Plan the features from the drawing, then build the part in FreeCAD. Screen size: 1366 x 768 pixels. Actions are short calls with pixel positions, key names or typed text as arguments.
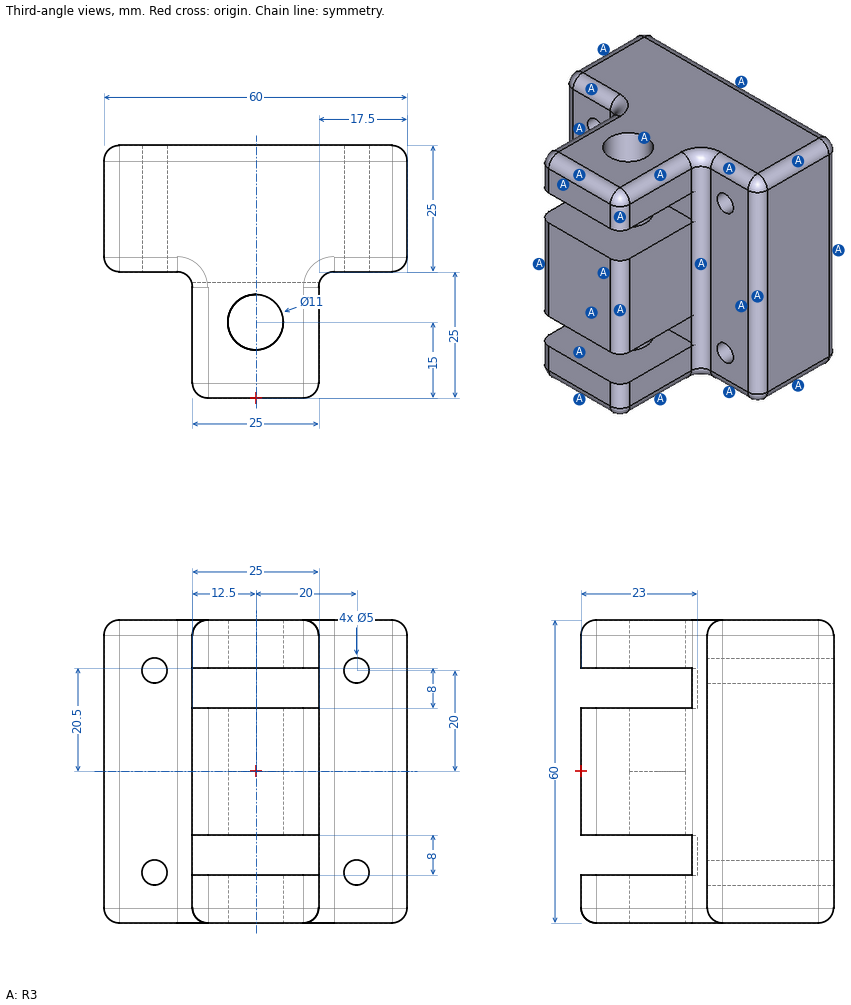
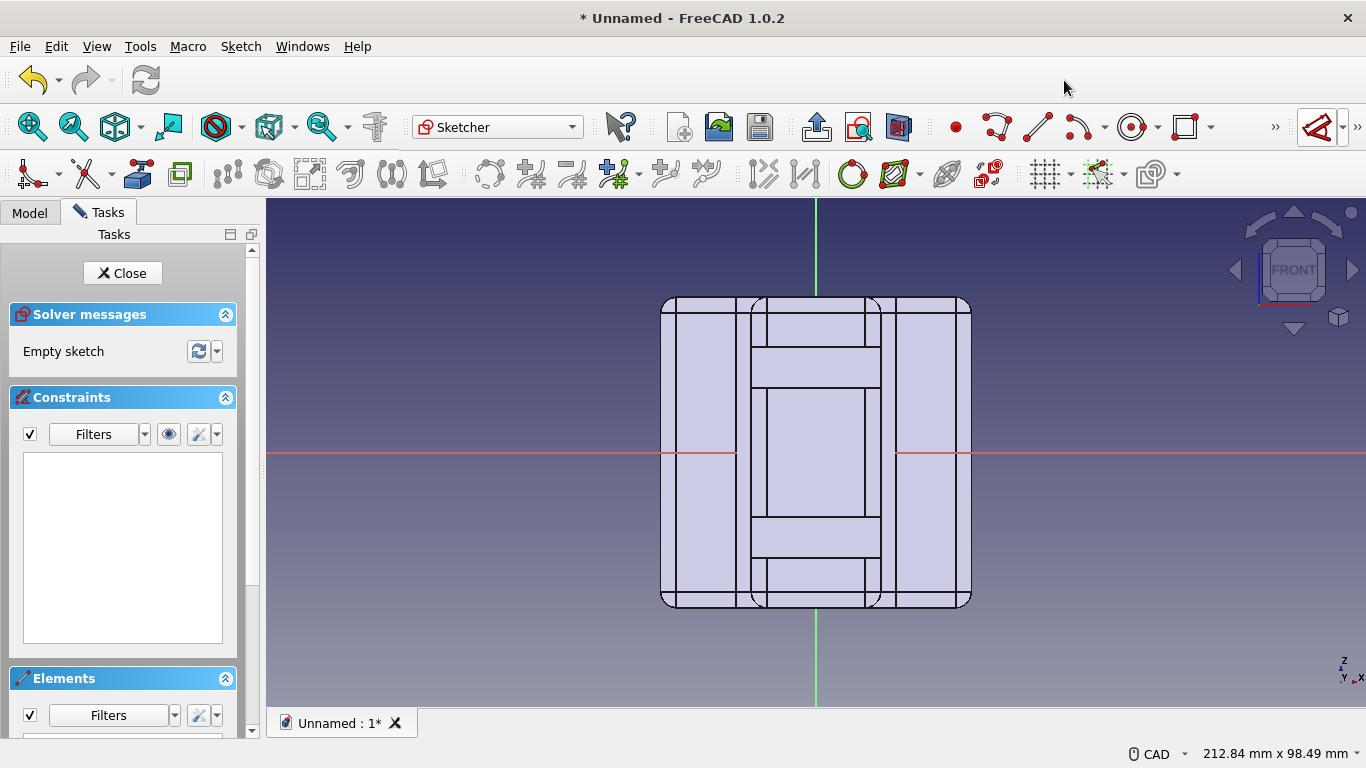
scroll(955, 453, up, 2)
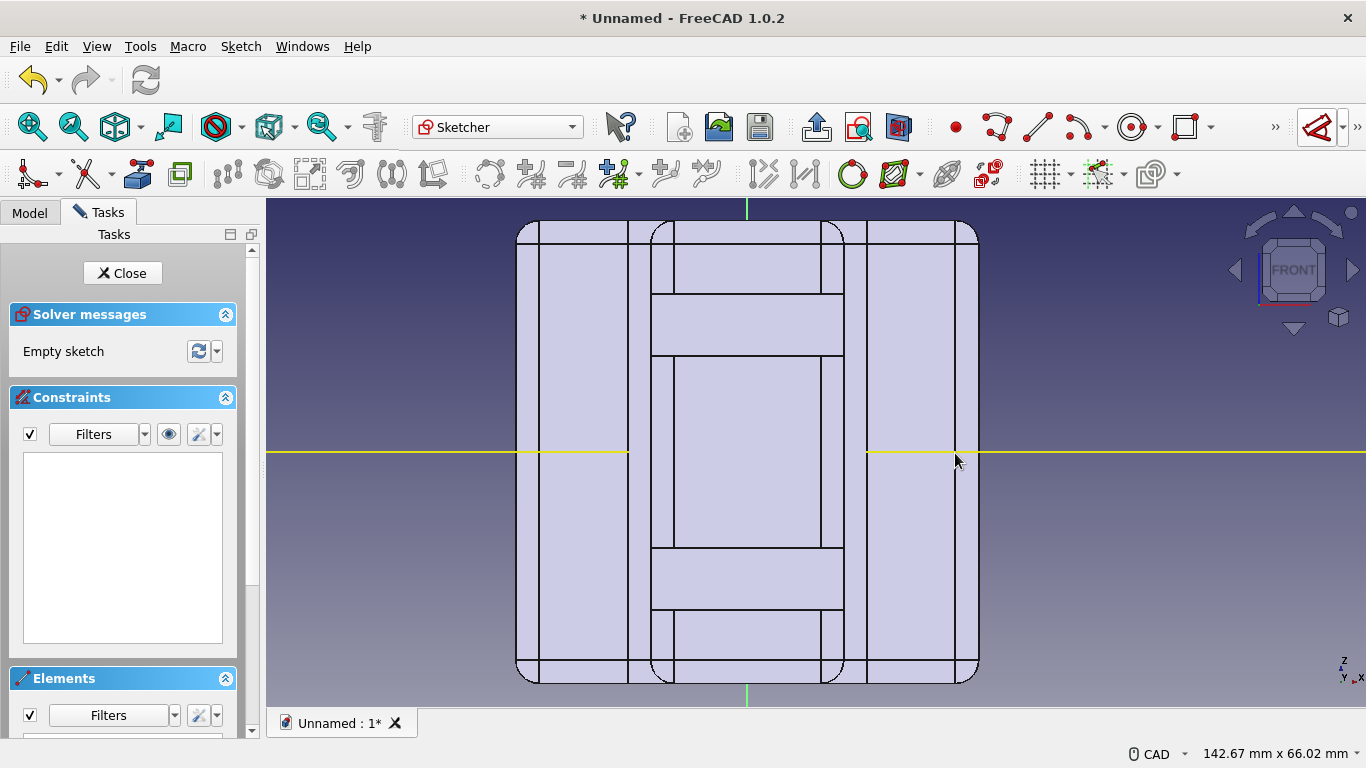
click(1132, 128)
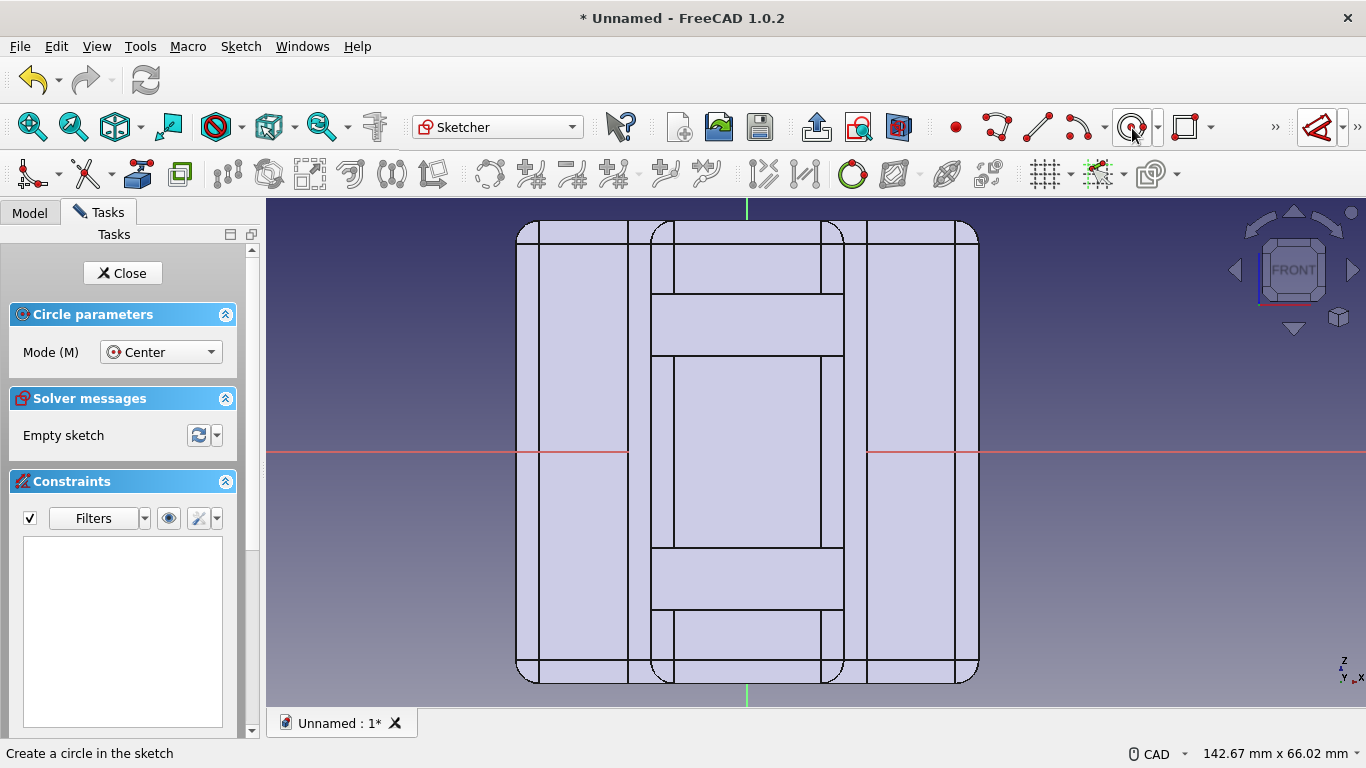
click(902, 298)
move(915, 284)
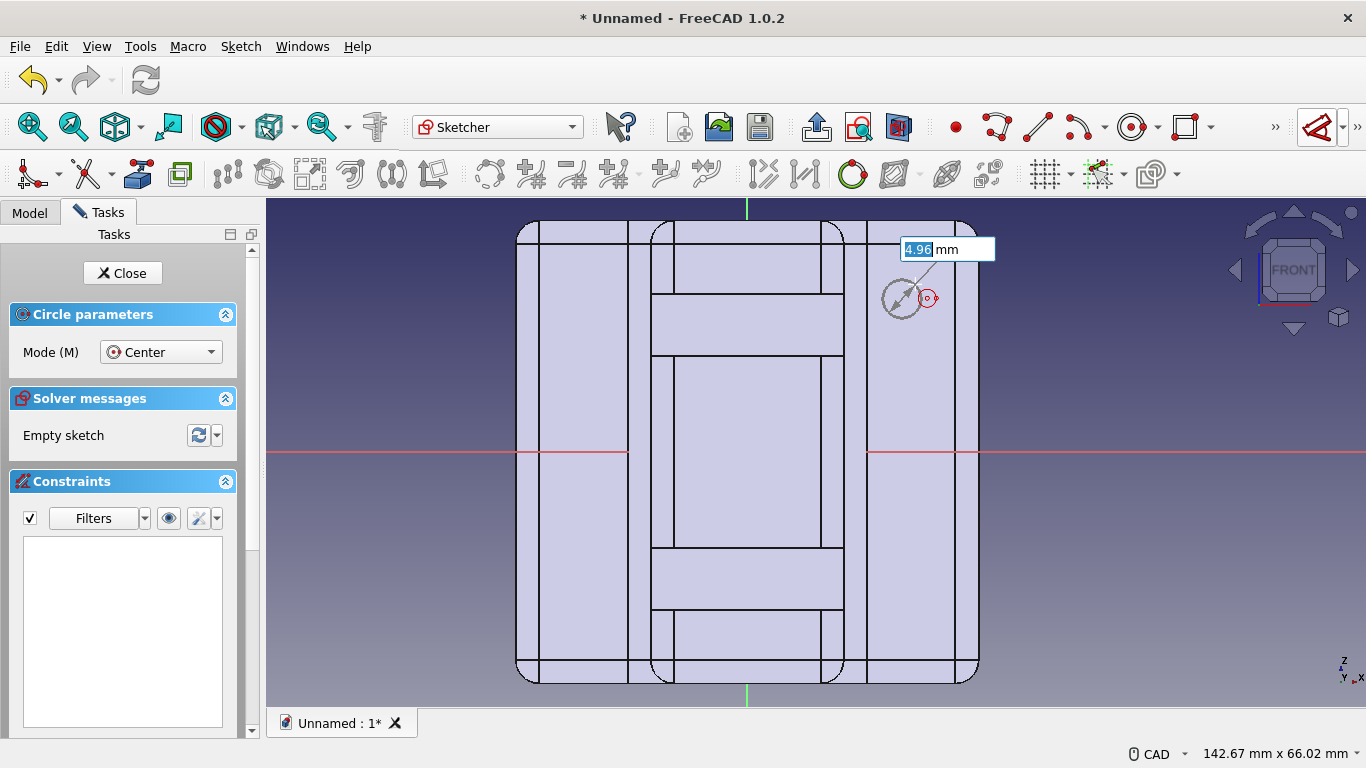
text(5)
key(Return)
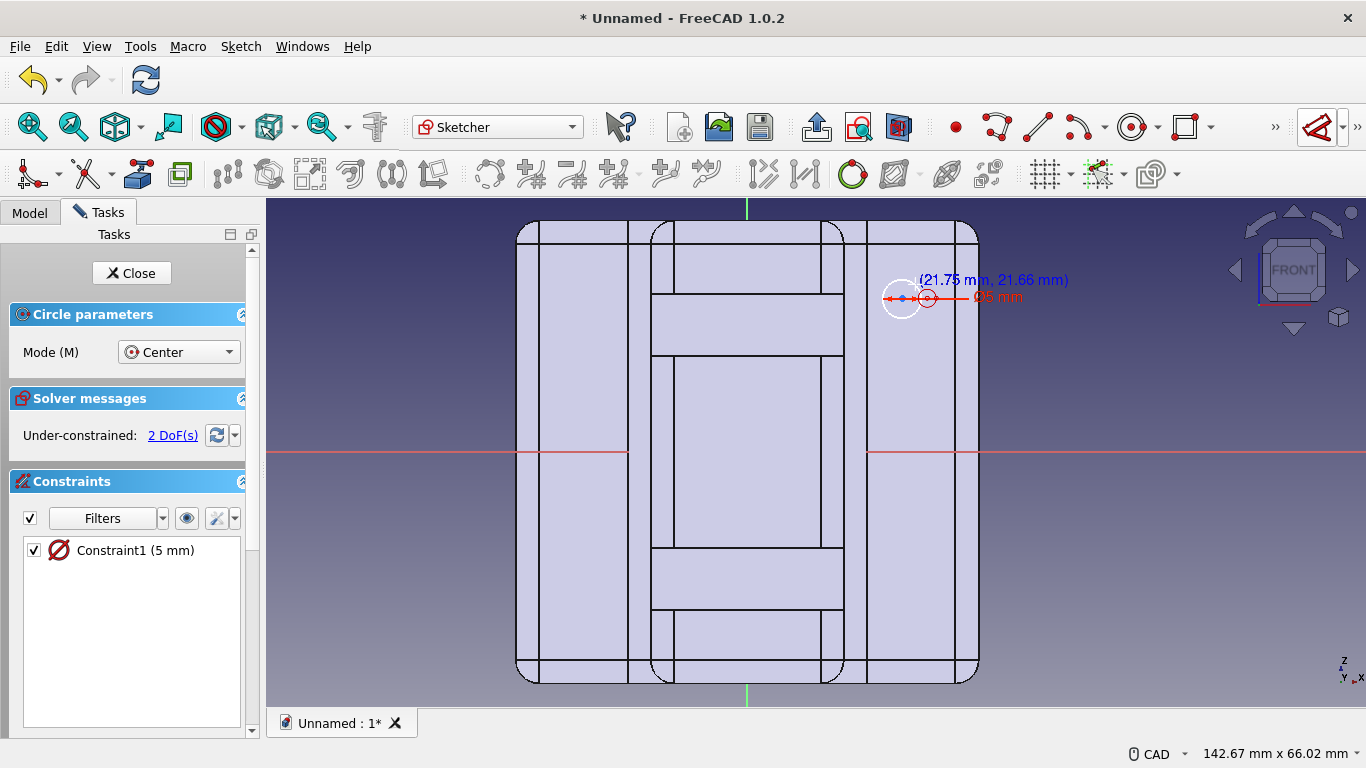
click(902, 606)
move(915, 593)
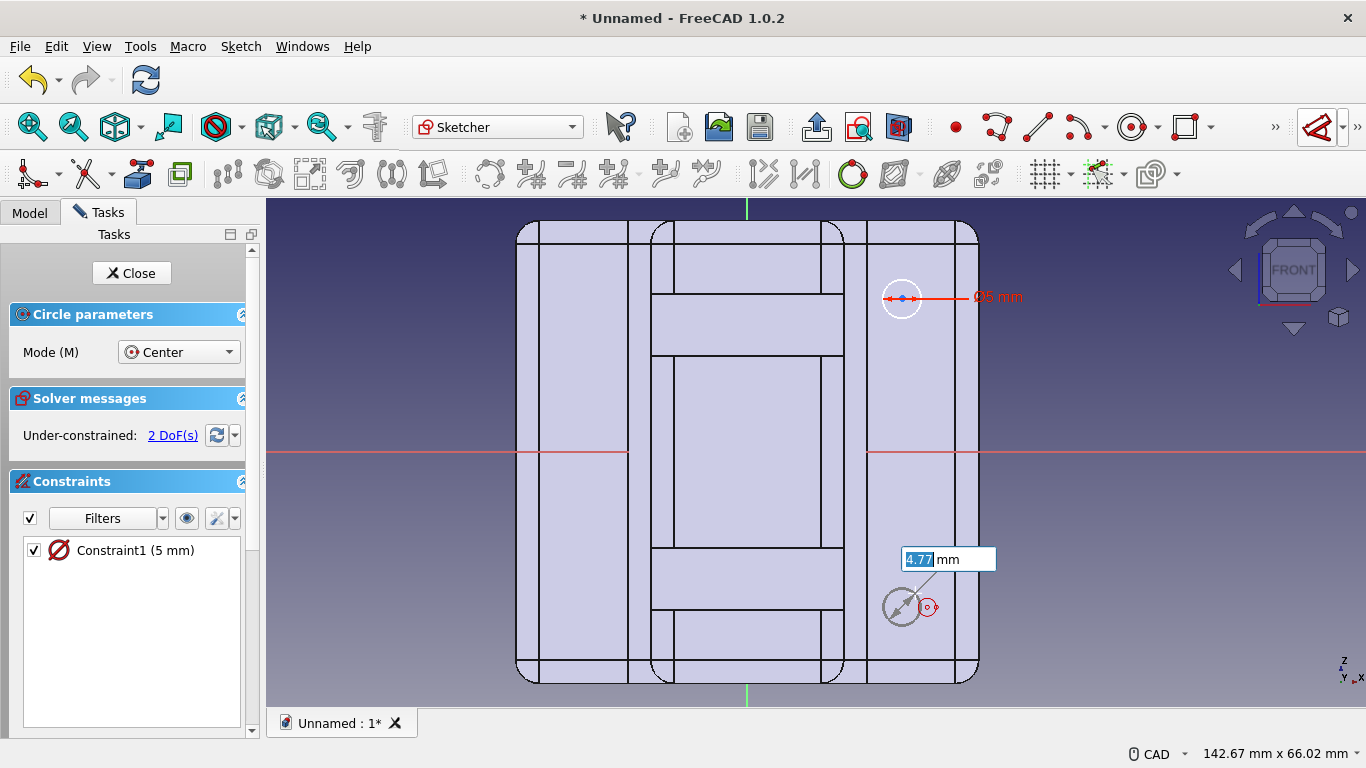
text(5)
key(Return)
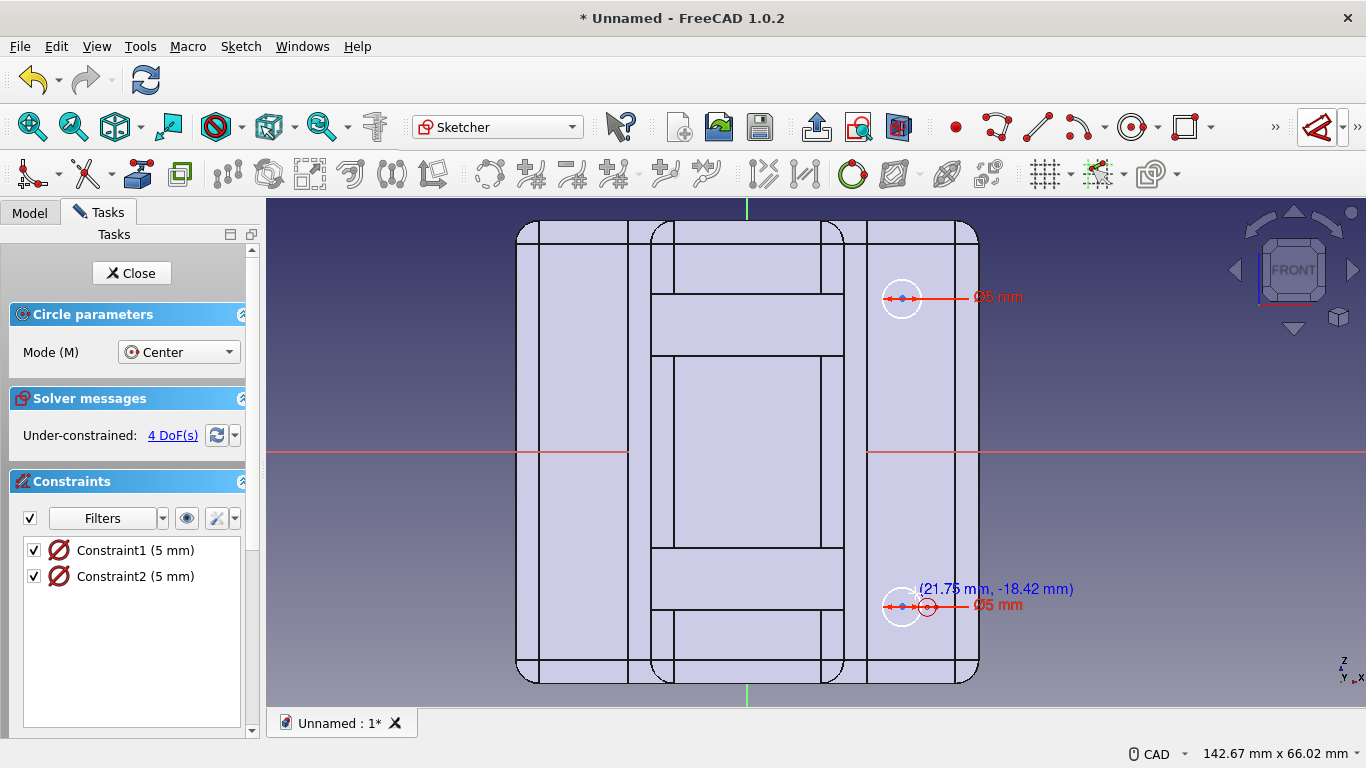
click(593, 606)
move(607, 593)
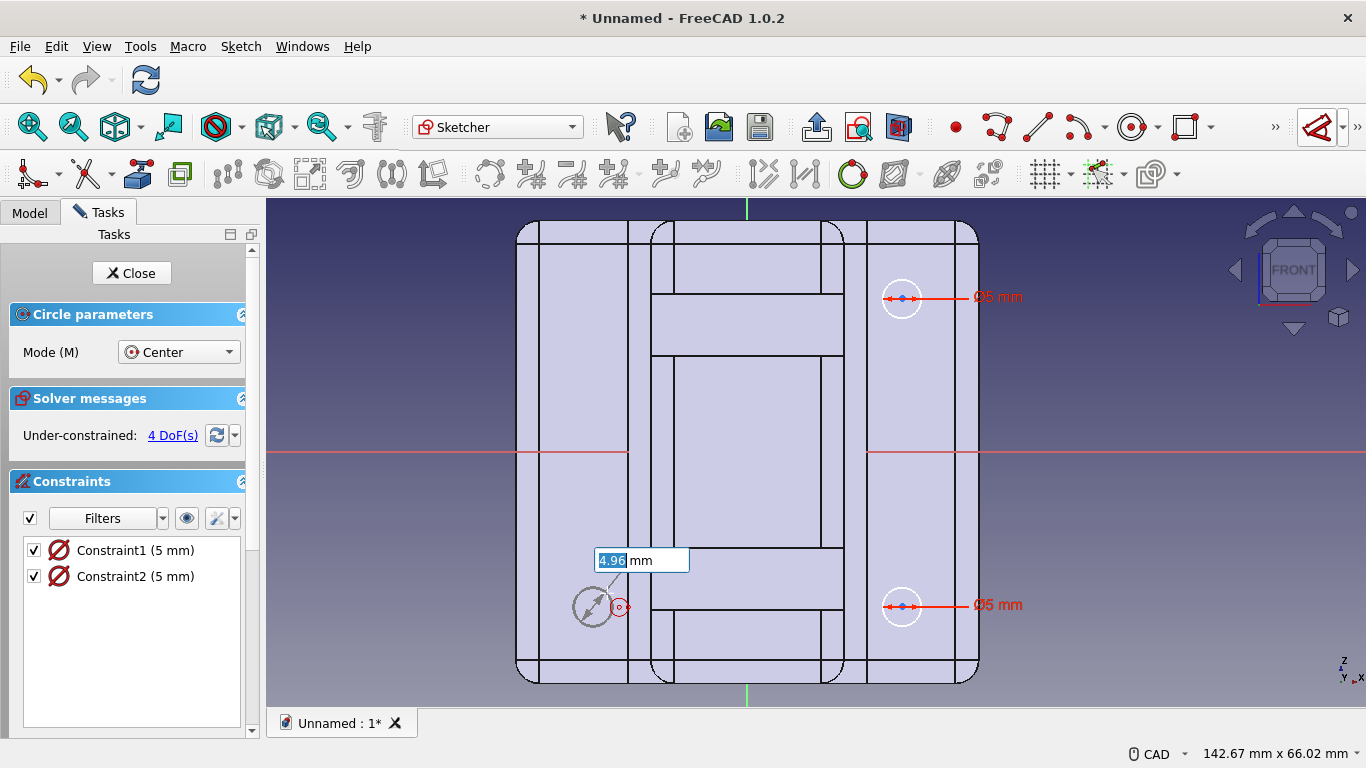
text(5)
key(Return)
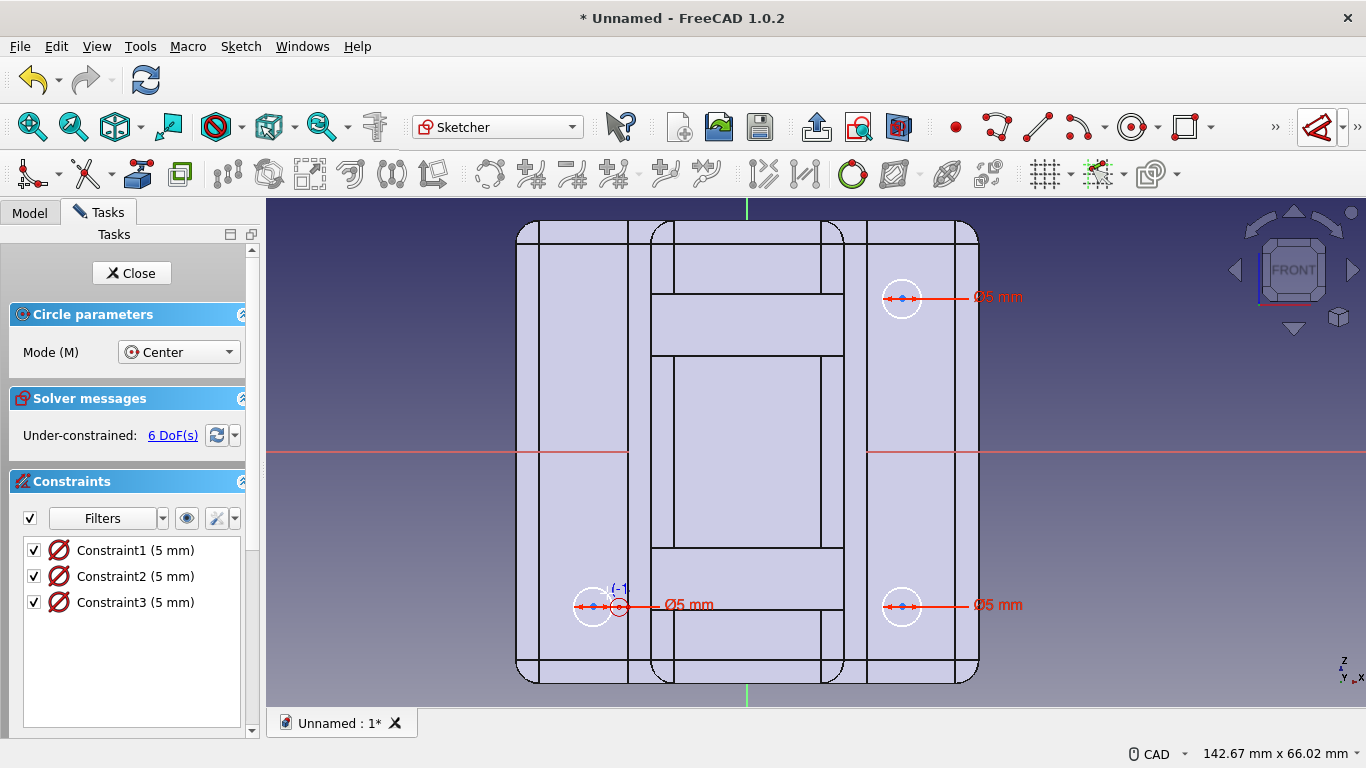
click(593, 298)
move(607, 284)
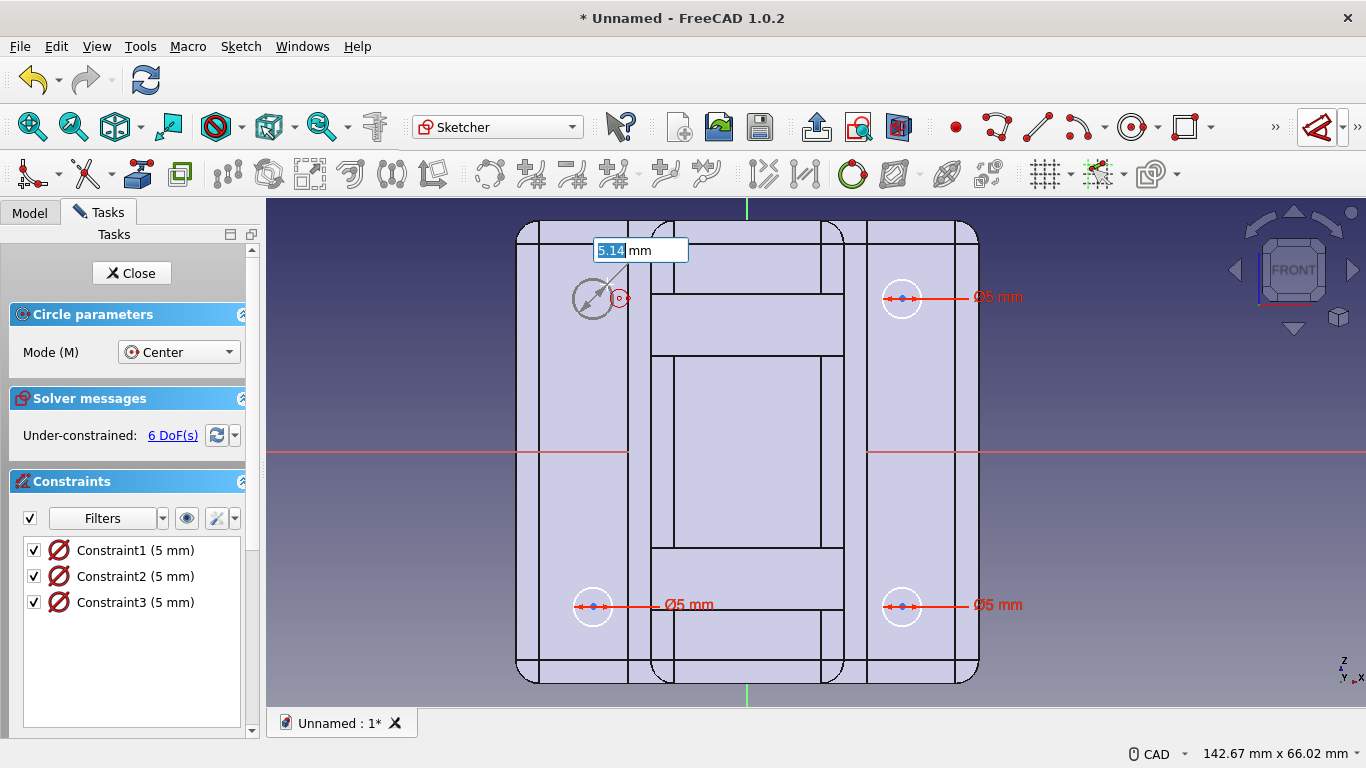
text(5)
key(Return)
key(Escape)